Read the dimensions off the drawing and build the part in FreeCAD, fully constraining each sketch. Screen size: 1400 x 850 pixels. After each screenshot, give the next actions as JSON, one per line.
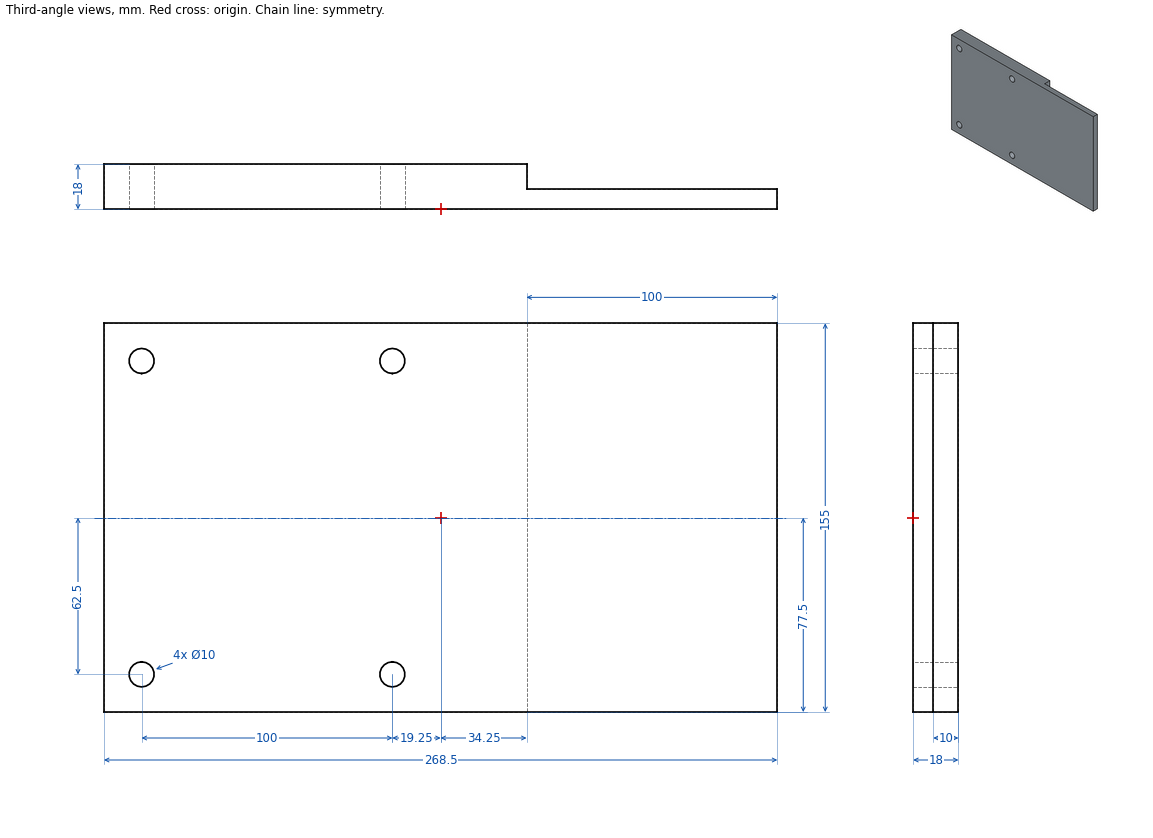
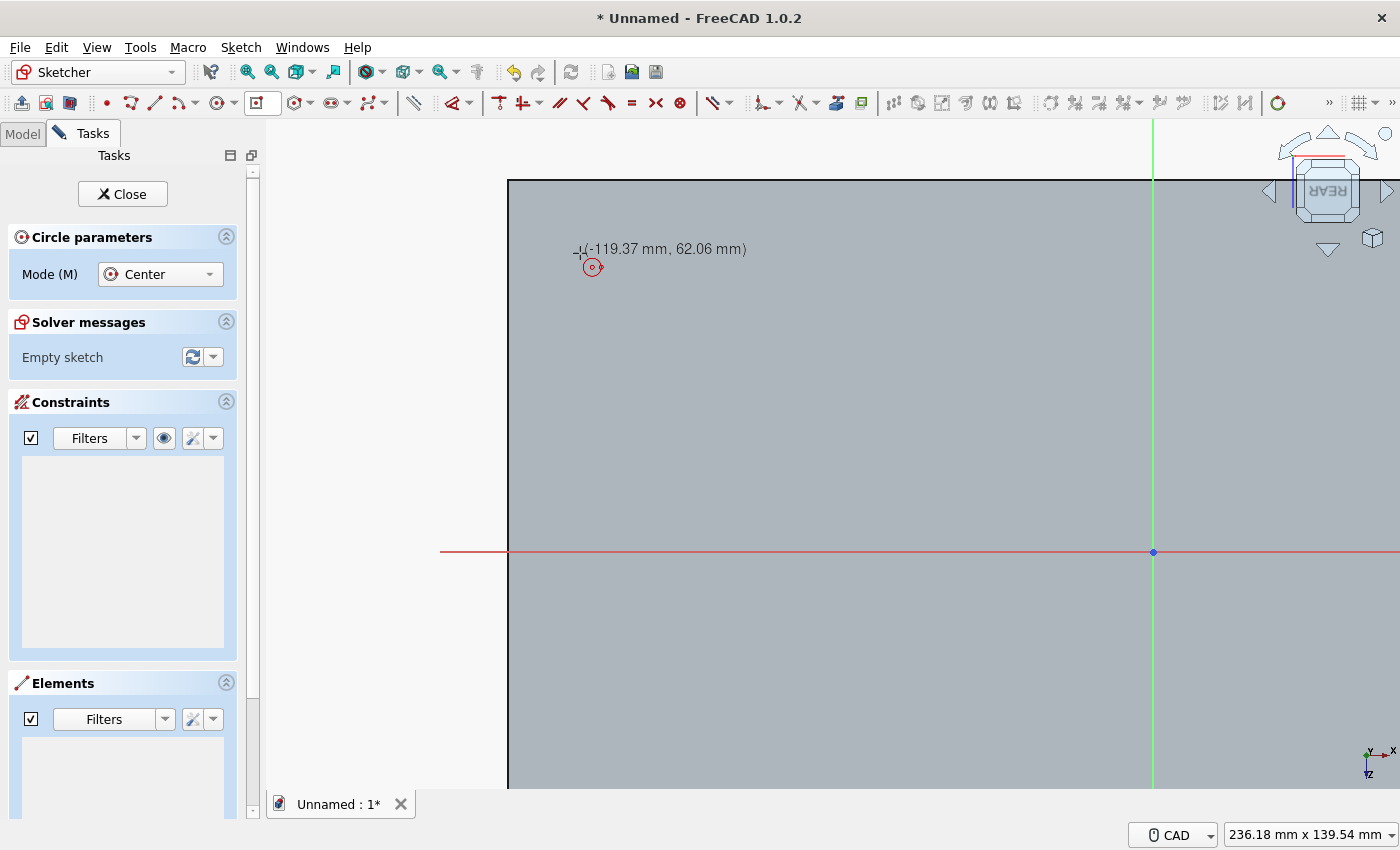
{"action": "left_click", "coordinate": [580, 252]}
{"action": "left_click", "coordinate": [597, 235]}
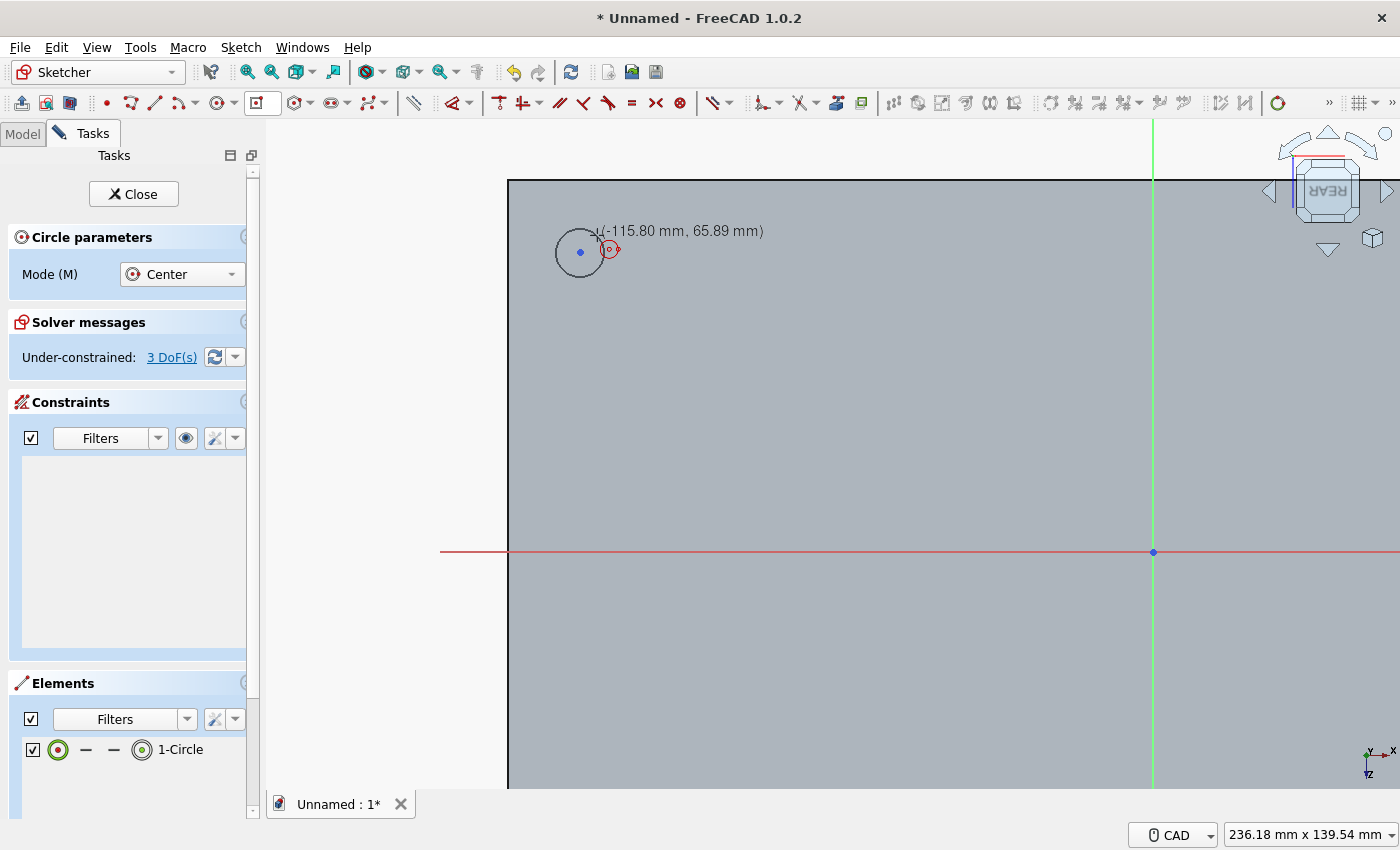
{"action": "left_click", "coordinate": [1061, 252]}
{"action": "left_click", "coordinate": [1078, 235]}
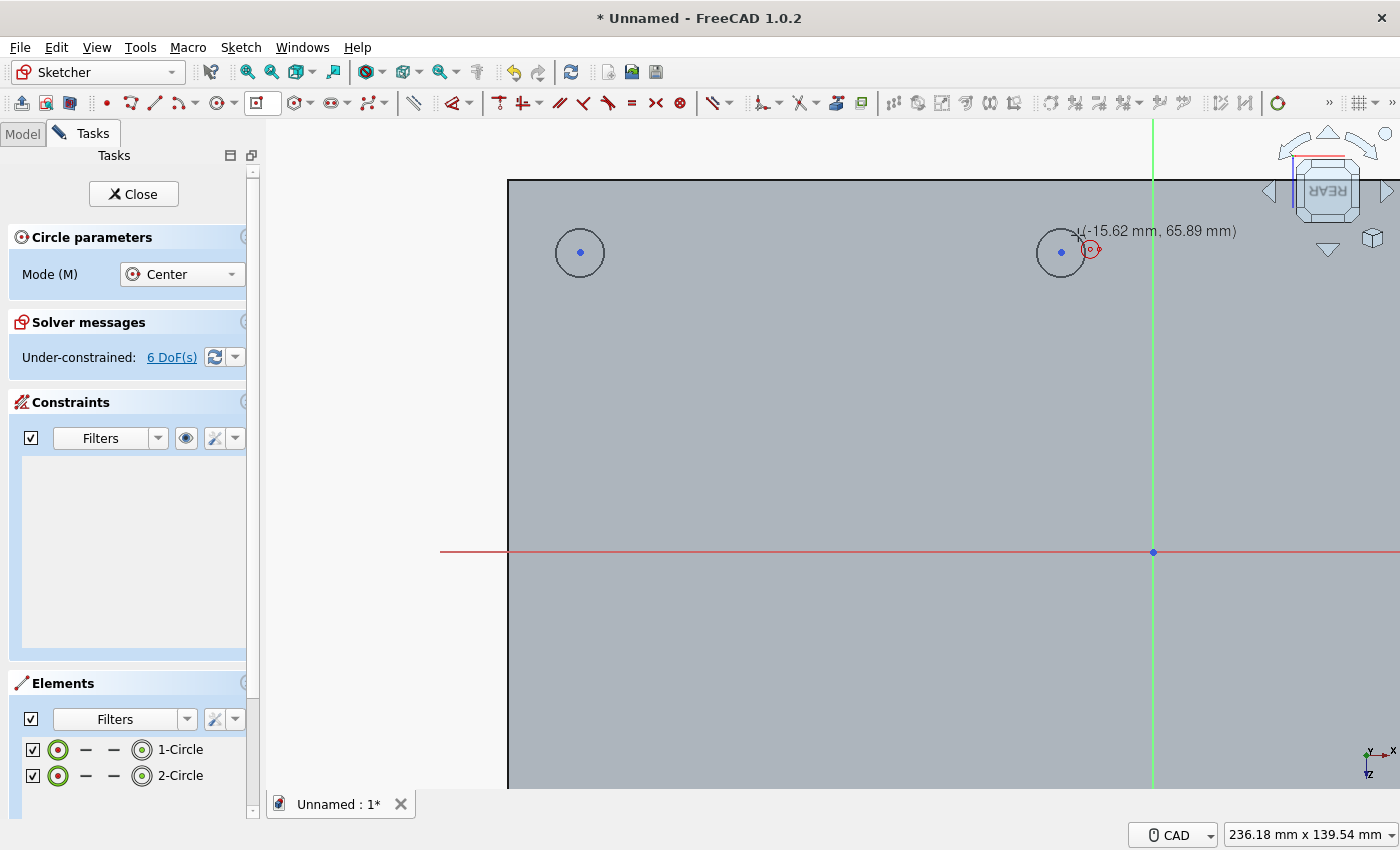
{"action": "scroll", "coordinate": [581, 254], "scroll_direction": "down", "scroll_amount": 2}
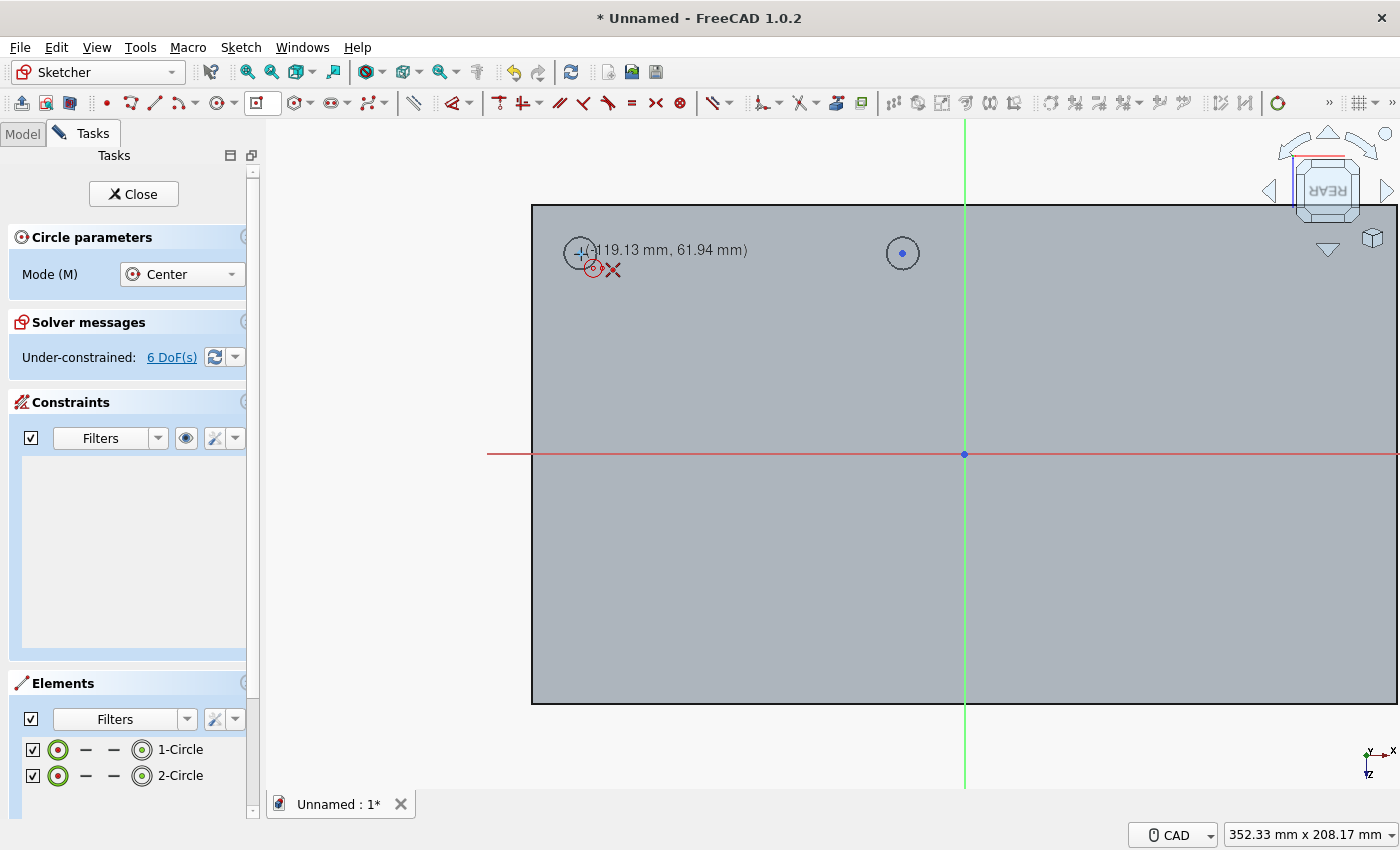
{"action": "scroll", "coordinate": [903, 655], "scroll_direction": "up", "scroll_amount": 2}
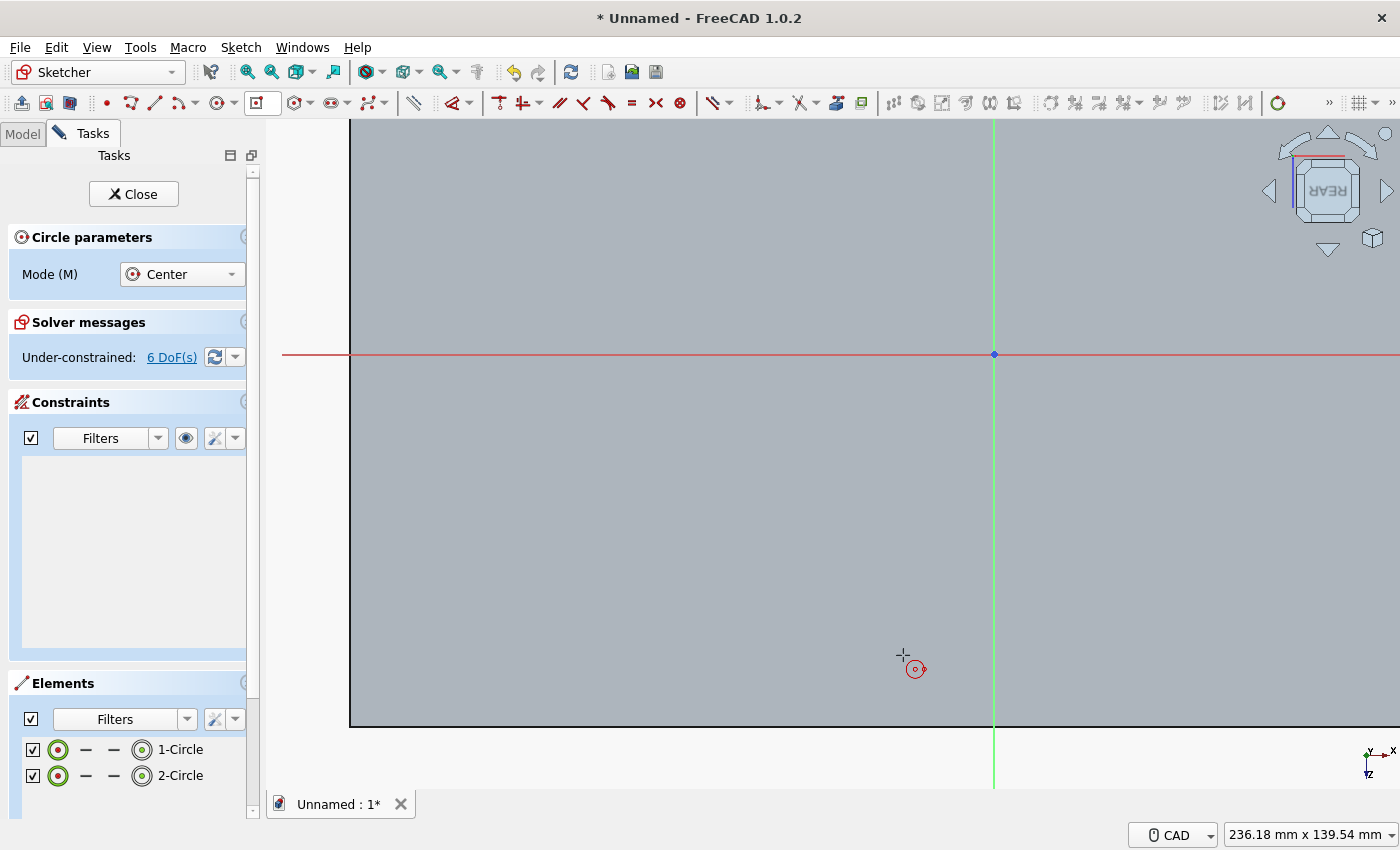
{"action": "left_click", "coordinate": [902, 655]}
{"action": "left_click", "coordinate": [919, 638]}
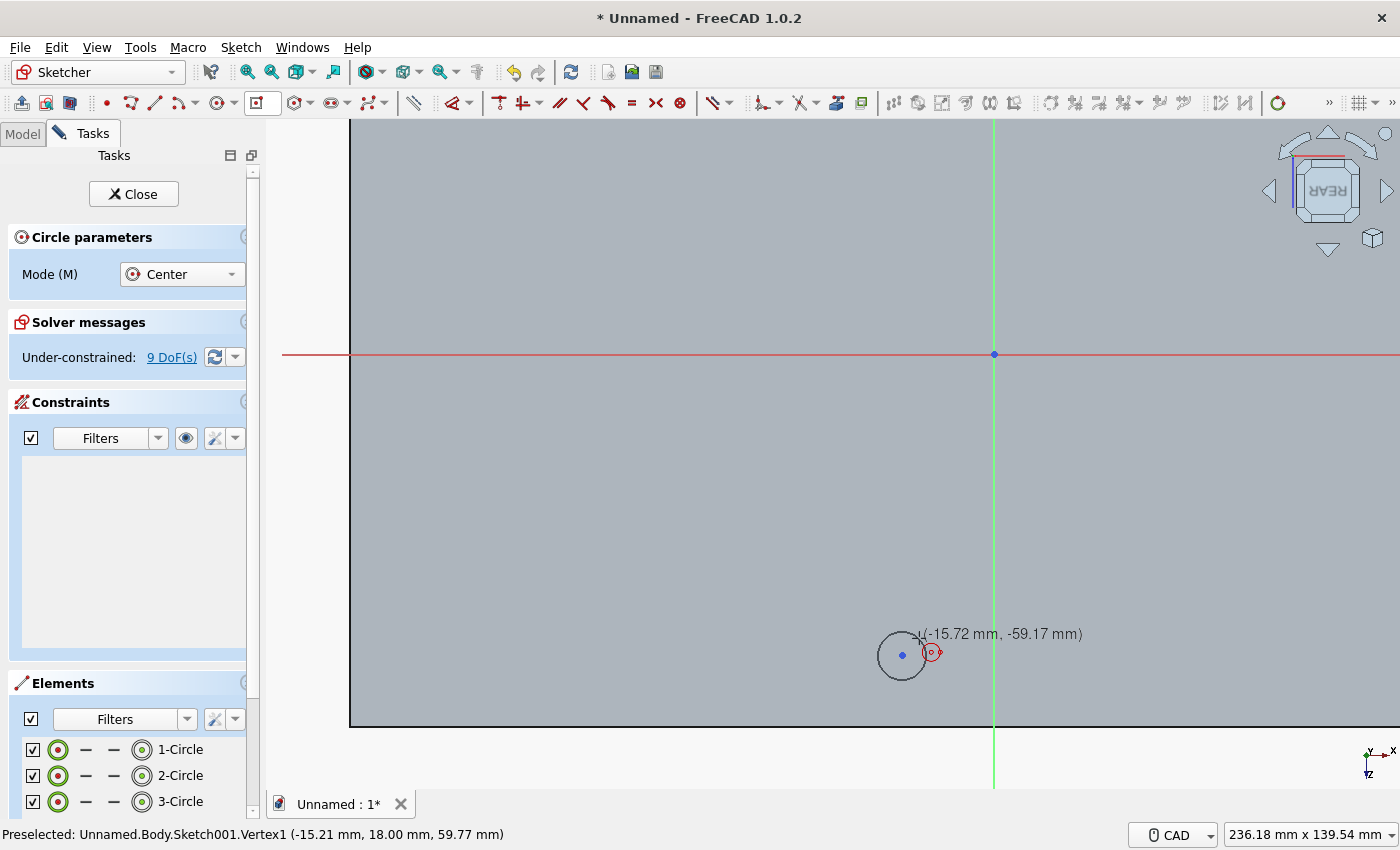
{"action": "left_click", "coordinate": [422, 655]}
{"action": "left_click", "coordinate": [439, 638]}
{"action": "key", "text": "Escape"}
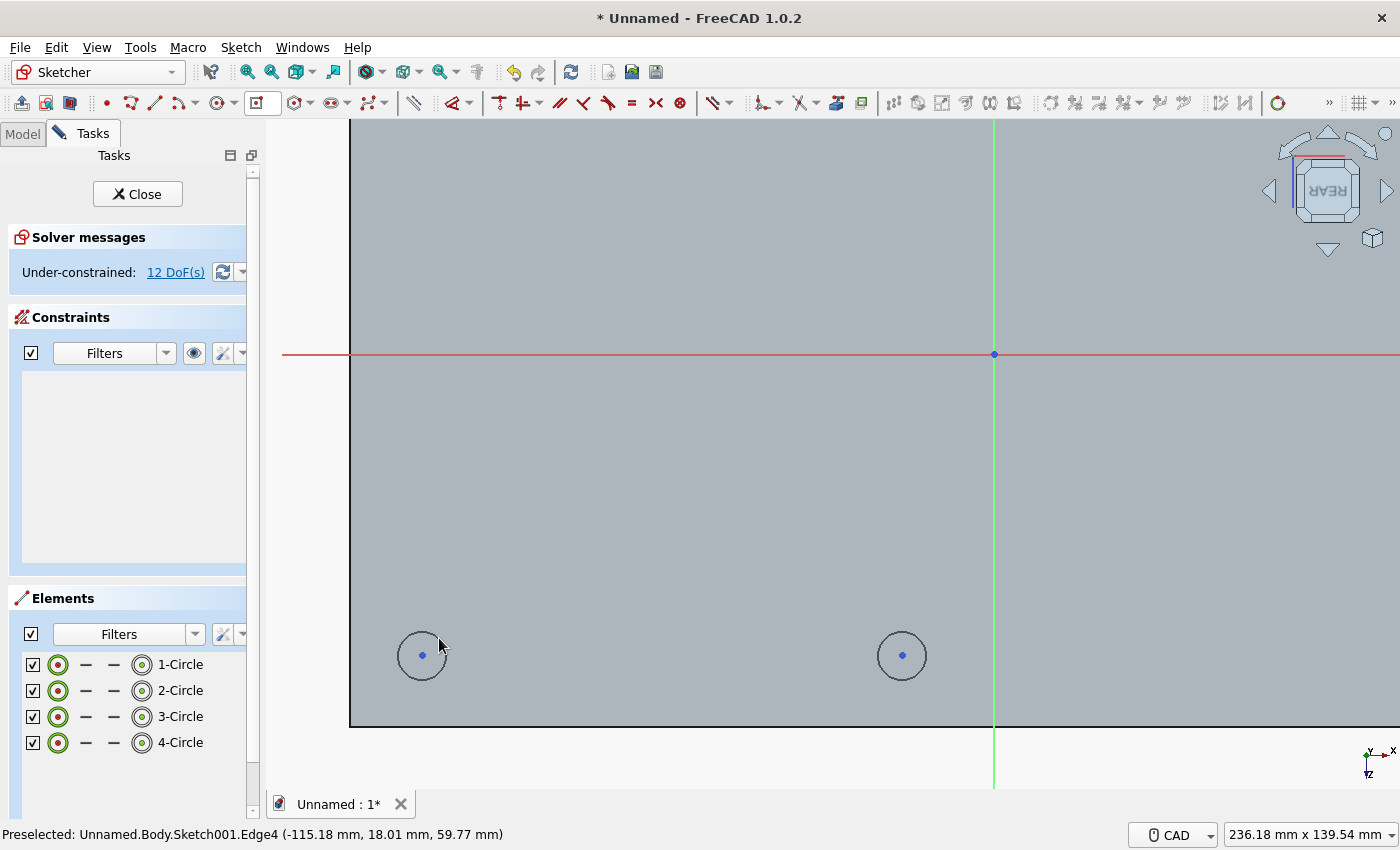
{"action": "scroll", "coordinate": [903, 656], "scroll_direction": "down", "scroll_amount": 2}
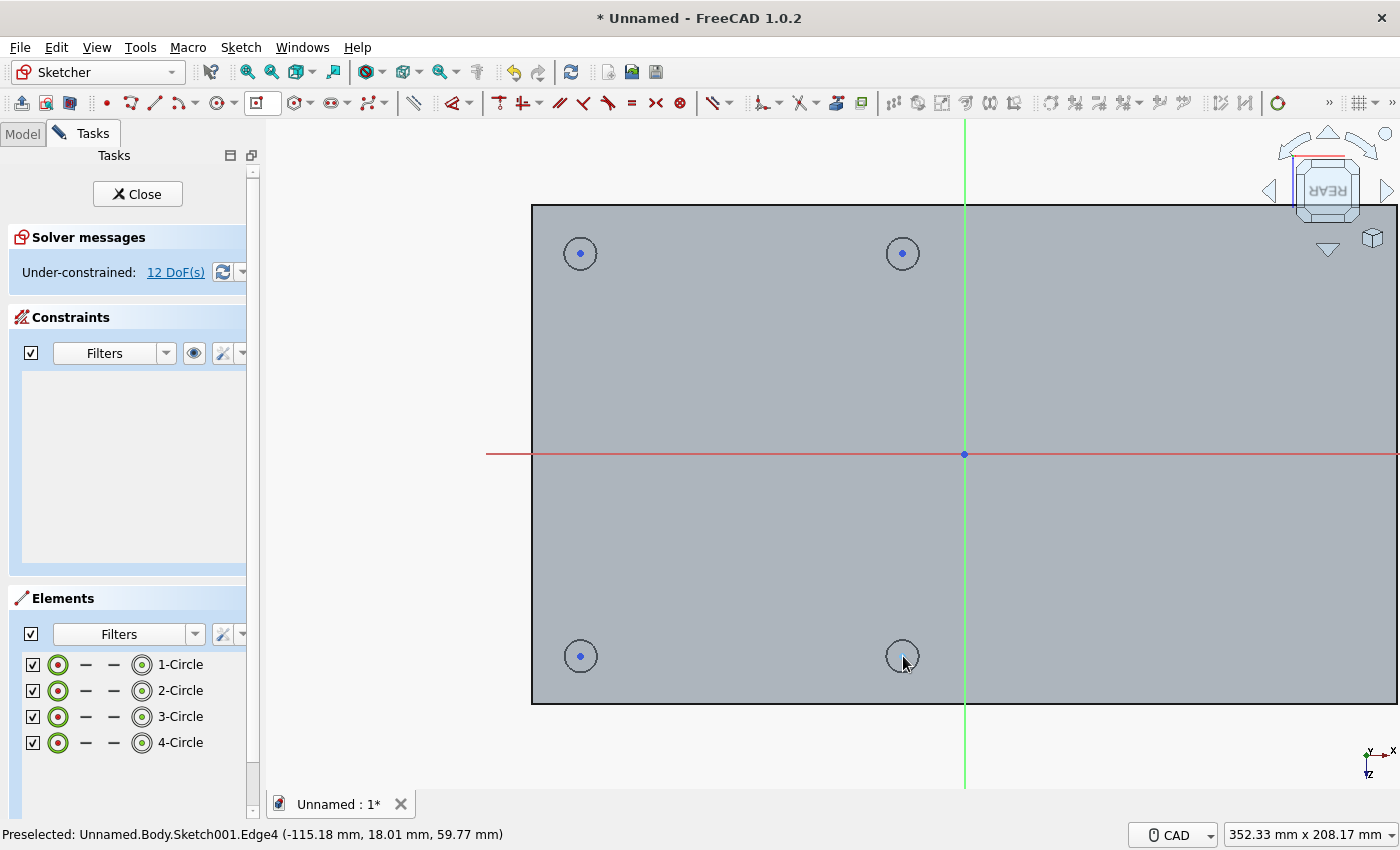
{"action": "left_click", "coordinate": [592, 242]}